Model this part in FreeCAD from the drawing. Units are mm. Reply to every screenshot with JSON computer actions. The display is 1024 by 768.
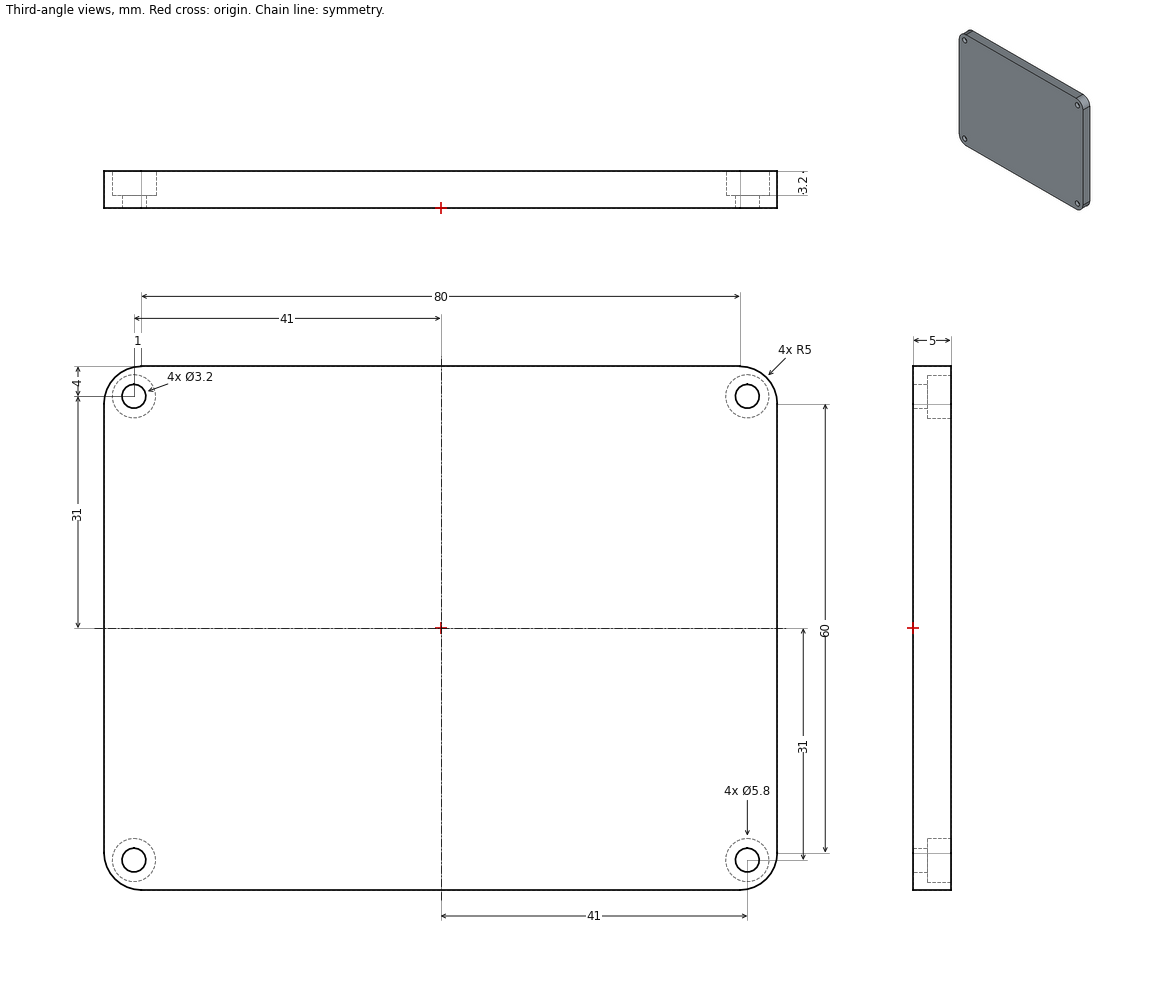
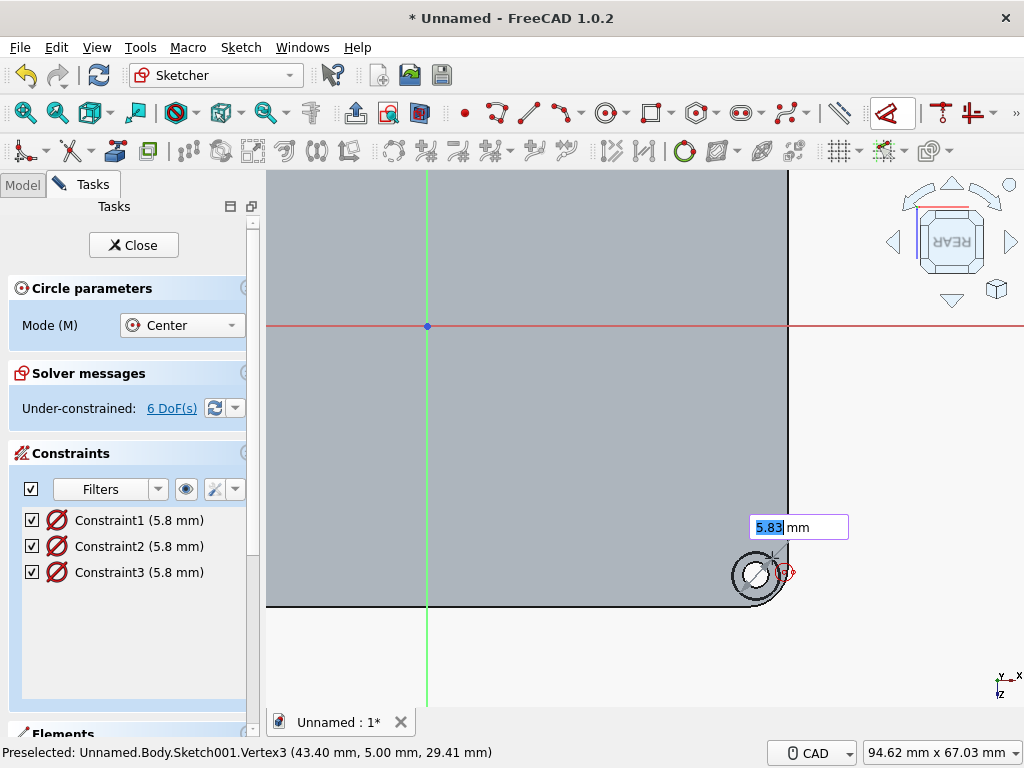
{"action": "type", "text": "5.8"}
{"action": "key", "text": "Return"}
{"action": "key", "text": "Escape"}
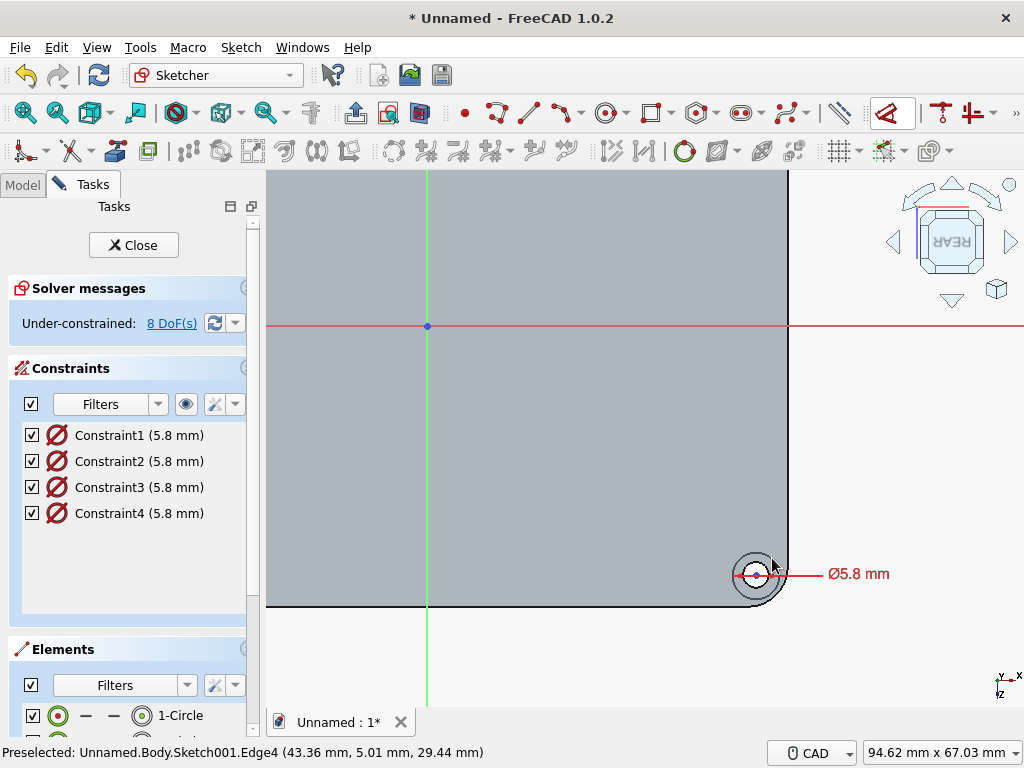
{"action": "scroll", "coordinate": [758, 575], "scroll_direction": "down", "scroll_amount": 3}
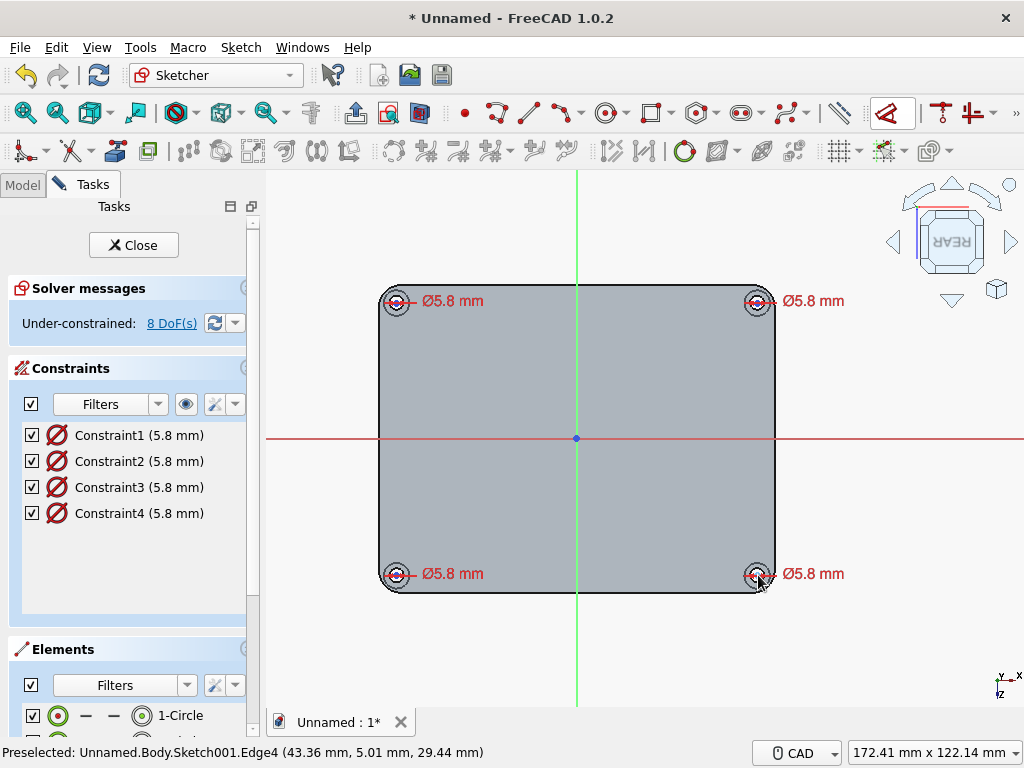
{"action": "left_click", "coordinate": [757, 303]}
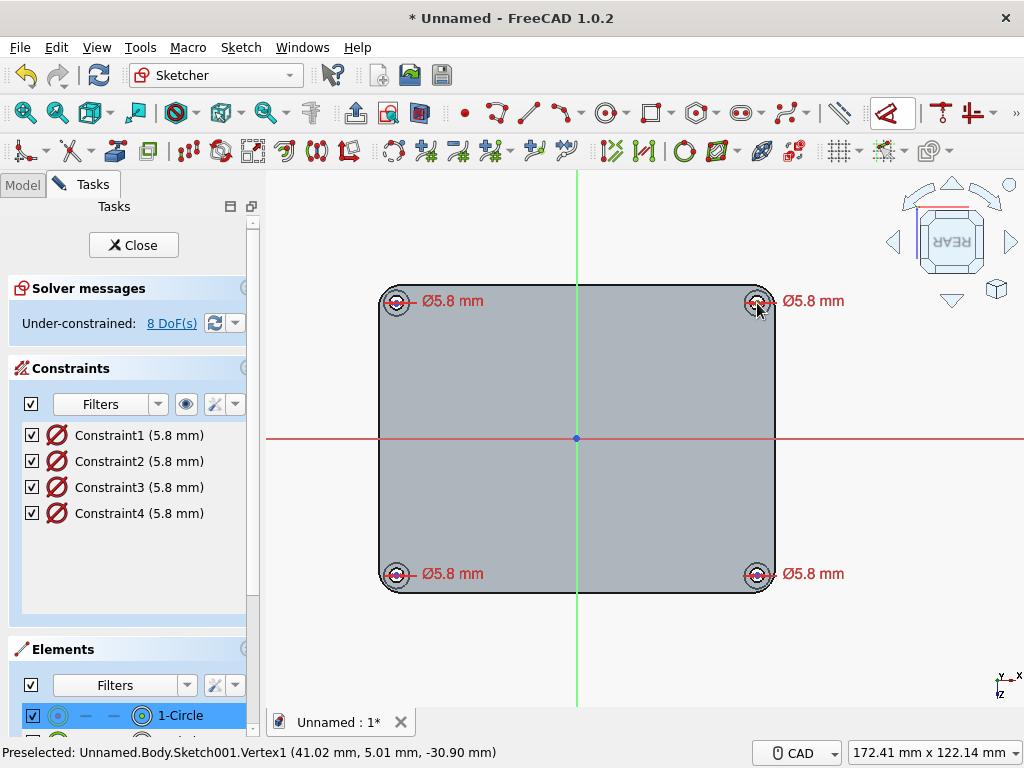
{"action": "left_click", "coordinate": [397, 303]}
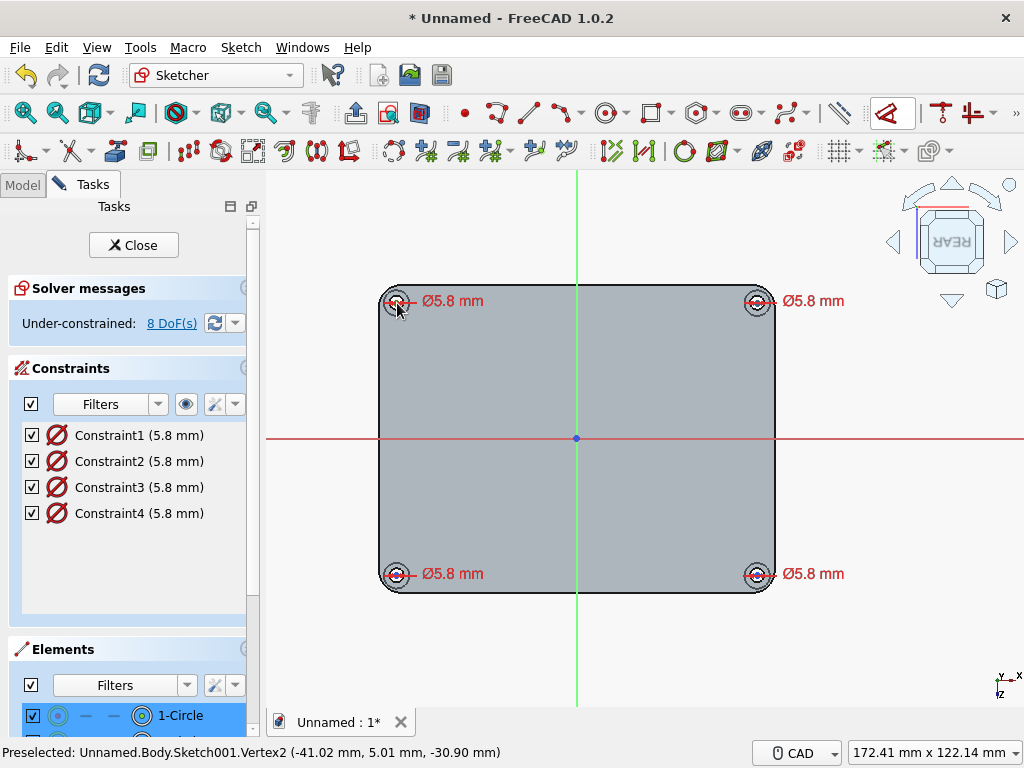
{"action": "key", "text": "h"}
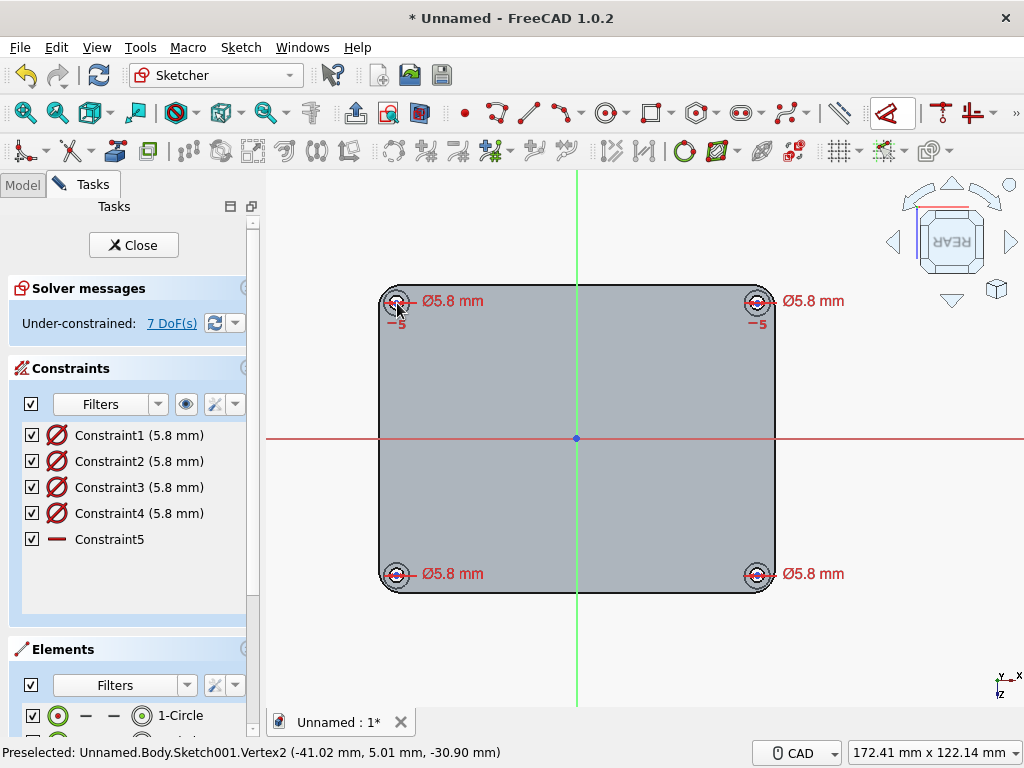
{"action": "left_click", "coordinate": [397, 303]}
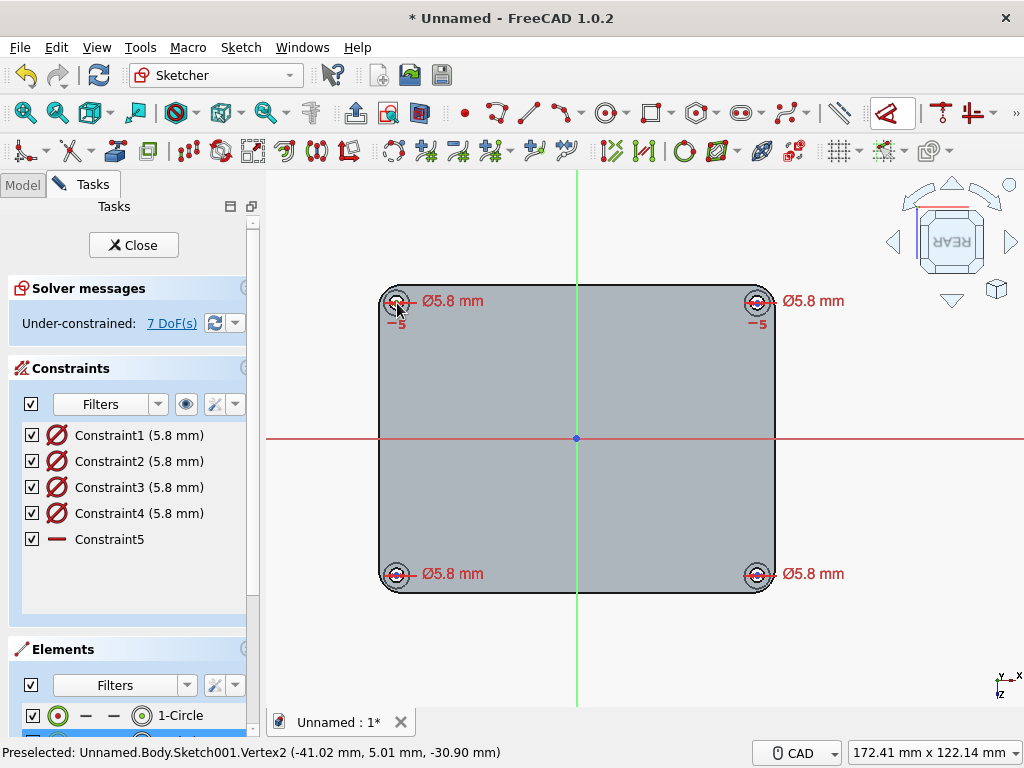
{"action": "left_click", "coordinate": [397, 576]}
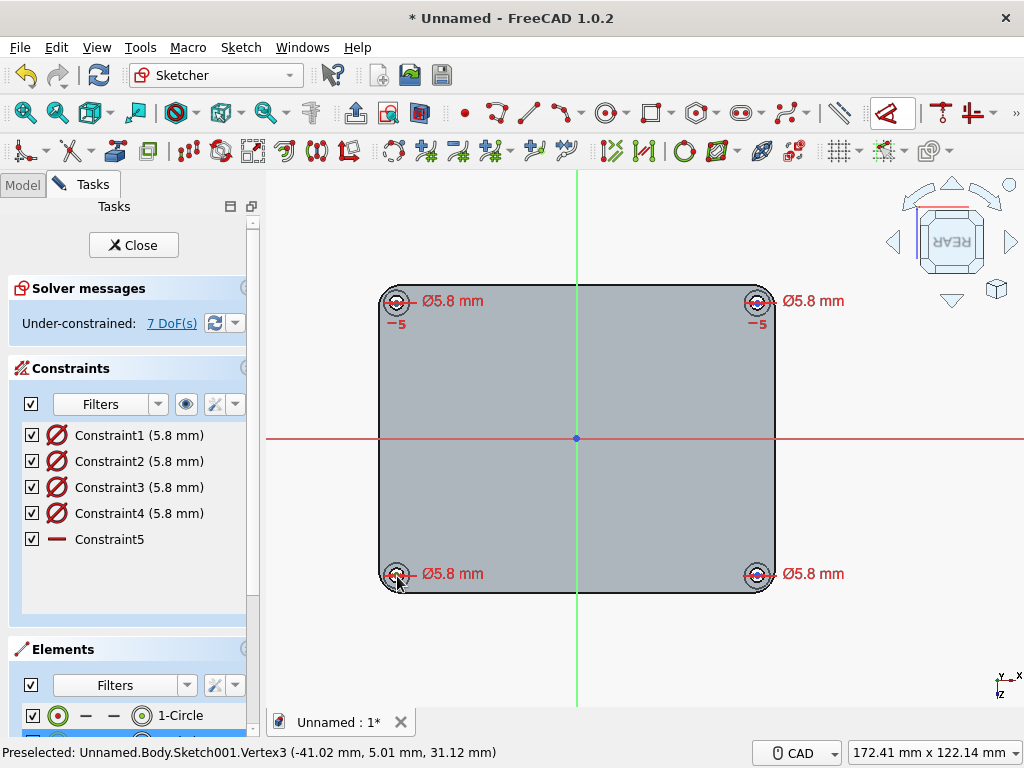
{"action": "key", "text": "v"}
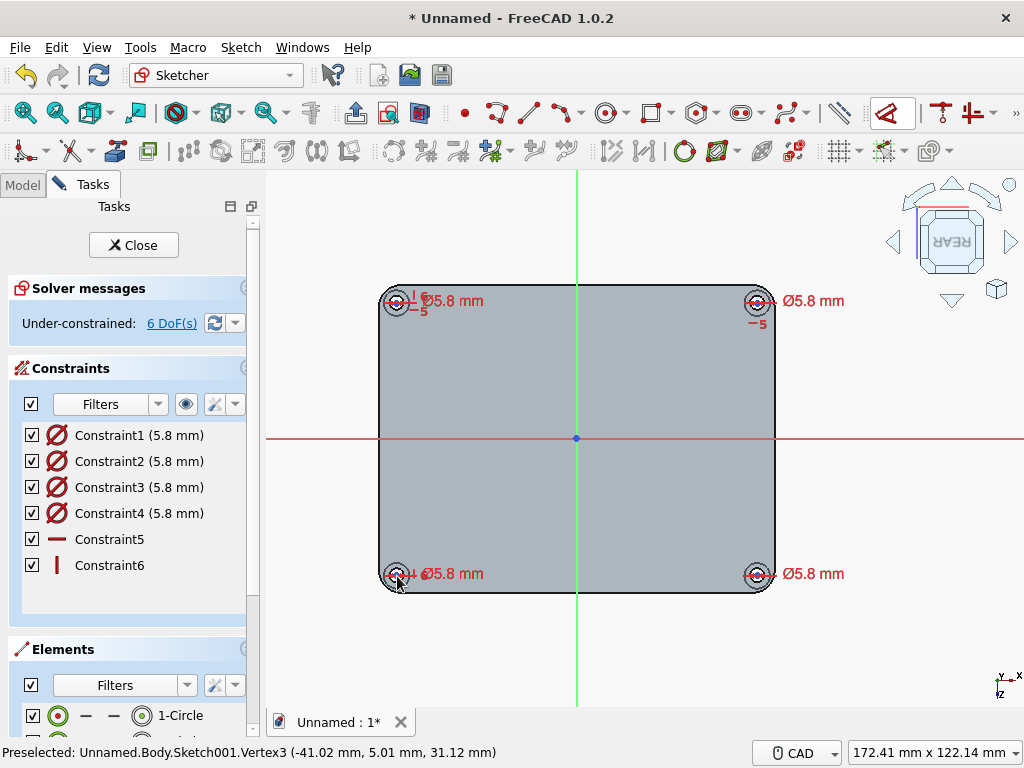
{"action": "left_click", "coordinate": [757, 303]}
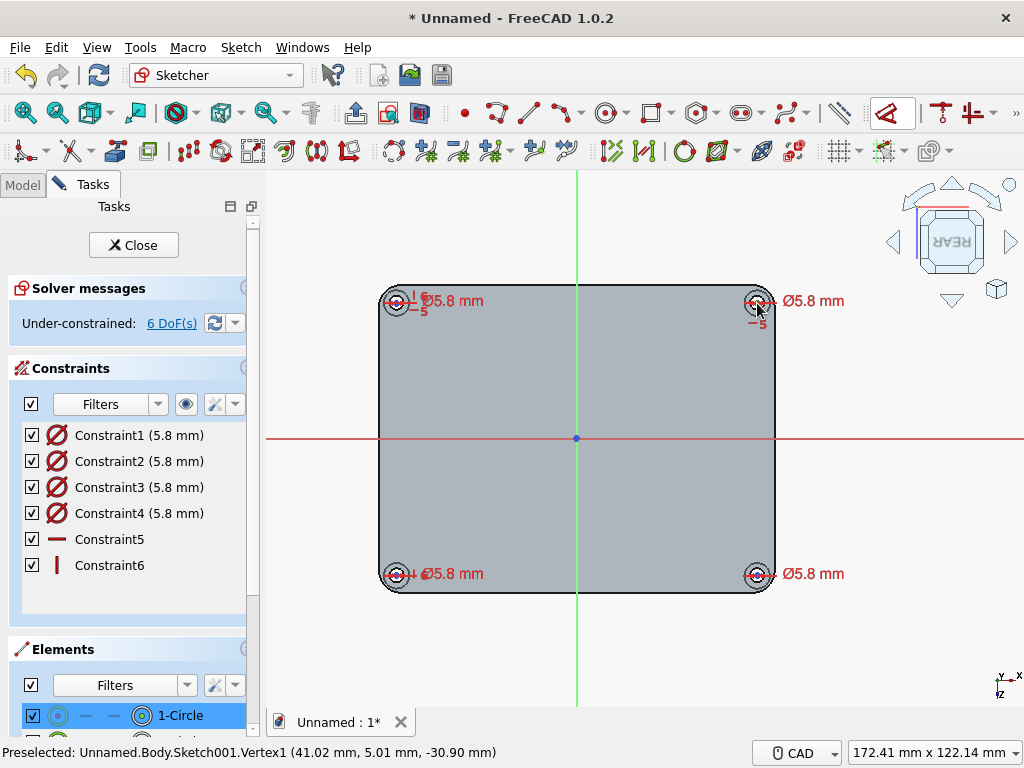
{"action": "left_click", "coordinate": [757, 576]}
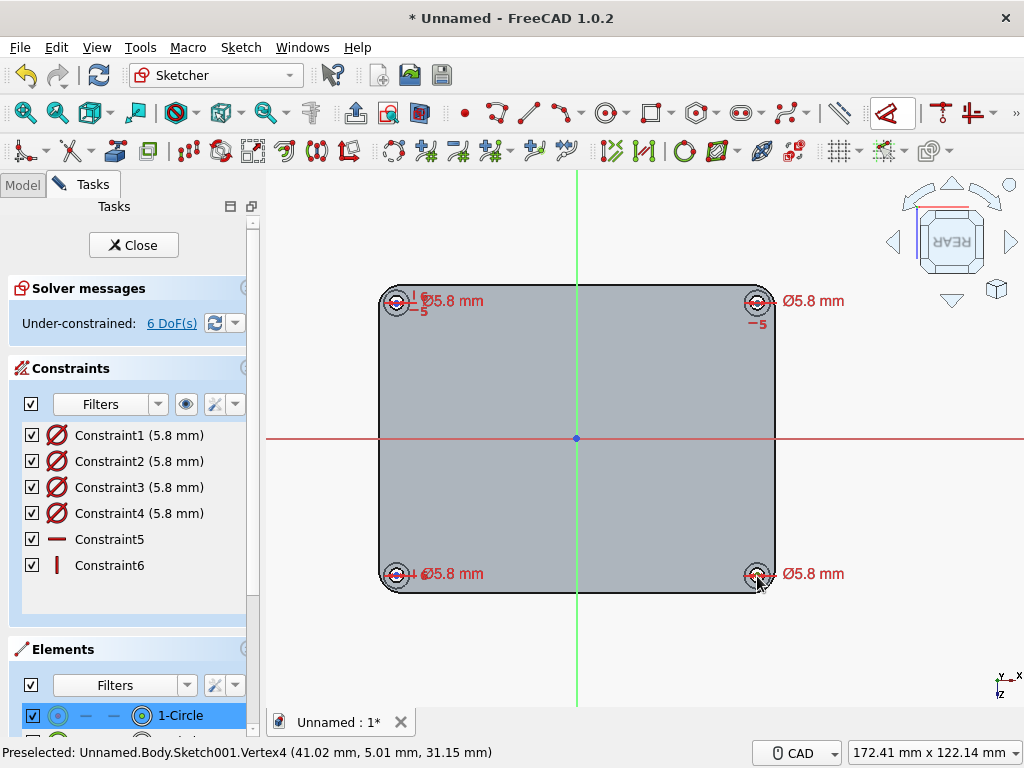
{"action": "key", "text": "v"}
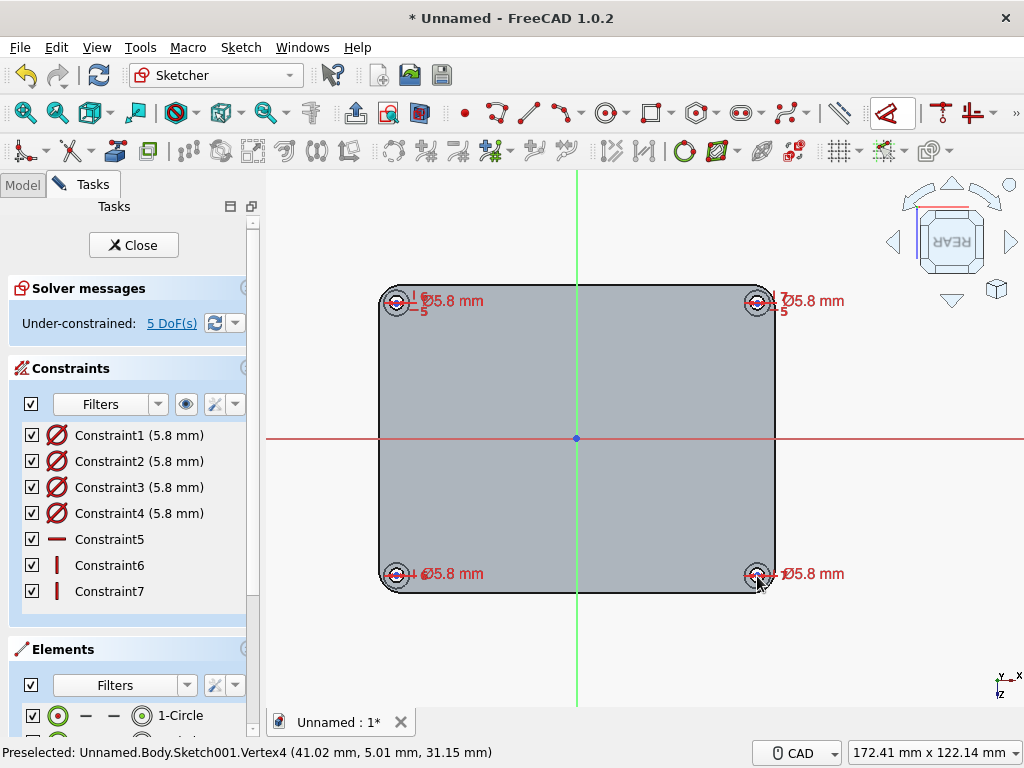
{"action": "left_click", "coordinate": [397, 576]}